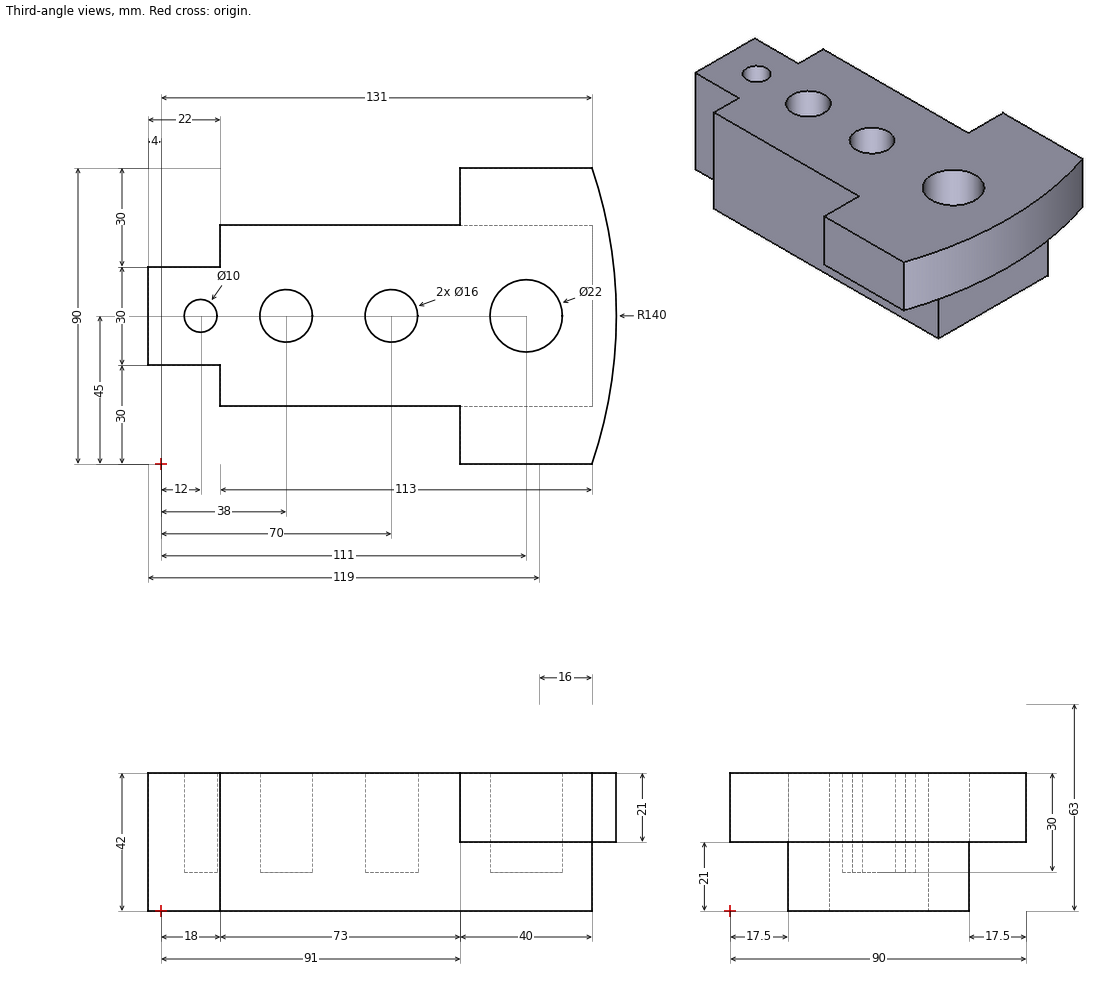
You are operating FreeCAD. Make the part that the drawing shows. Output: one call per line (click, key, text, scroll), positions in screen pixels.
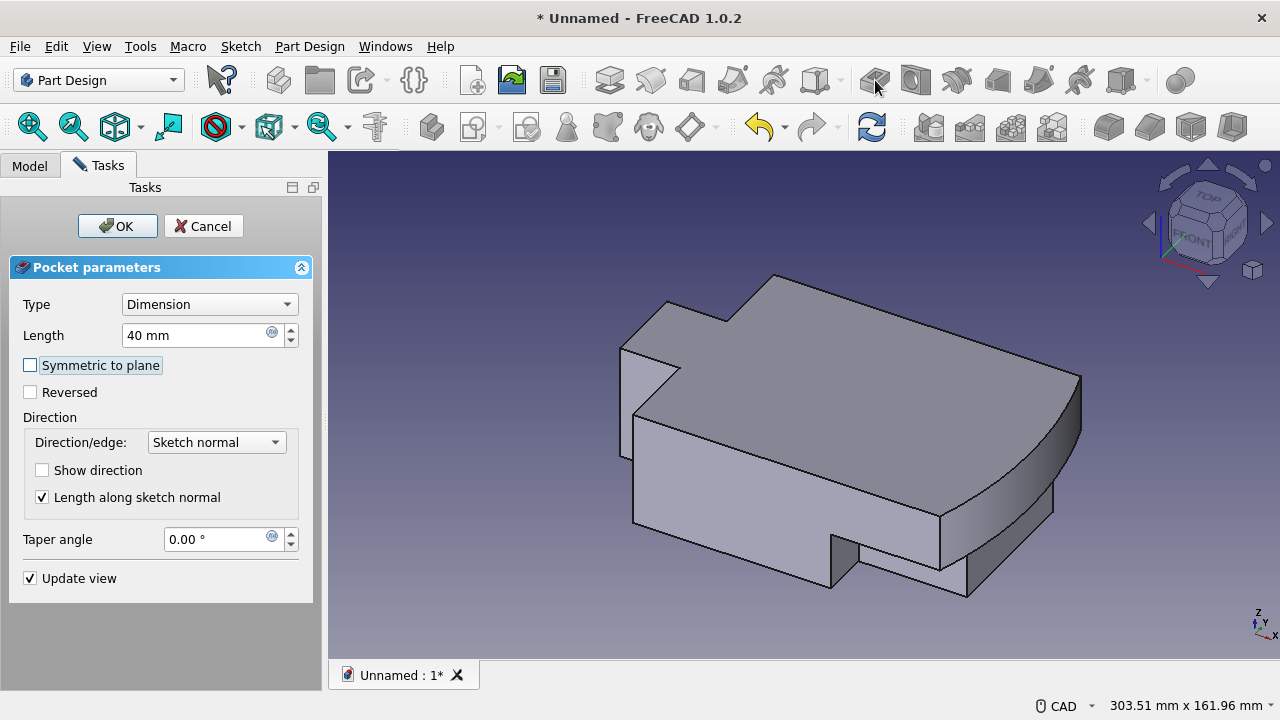
click(118, 226)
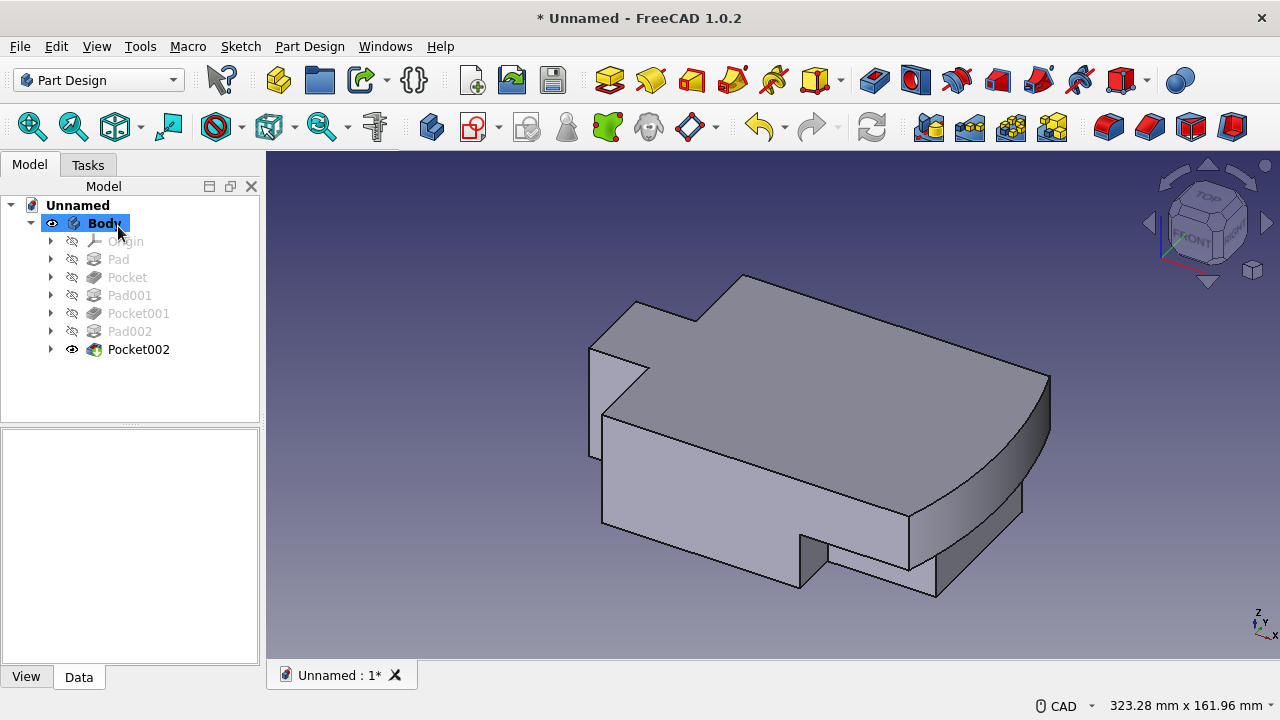
click(472, 128)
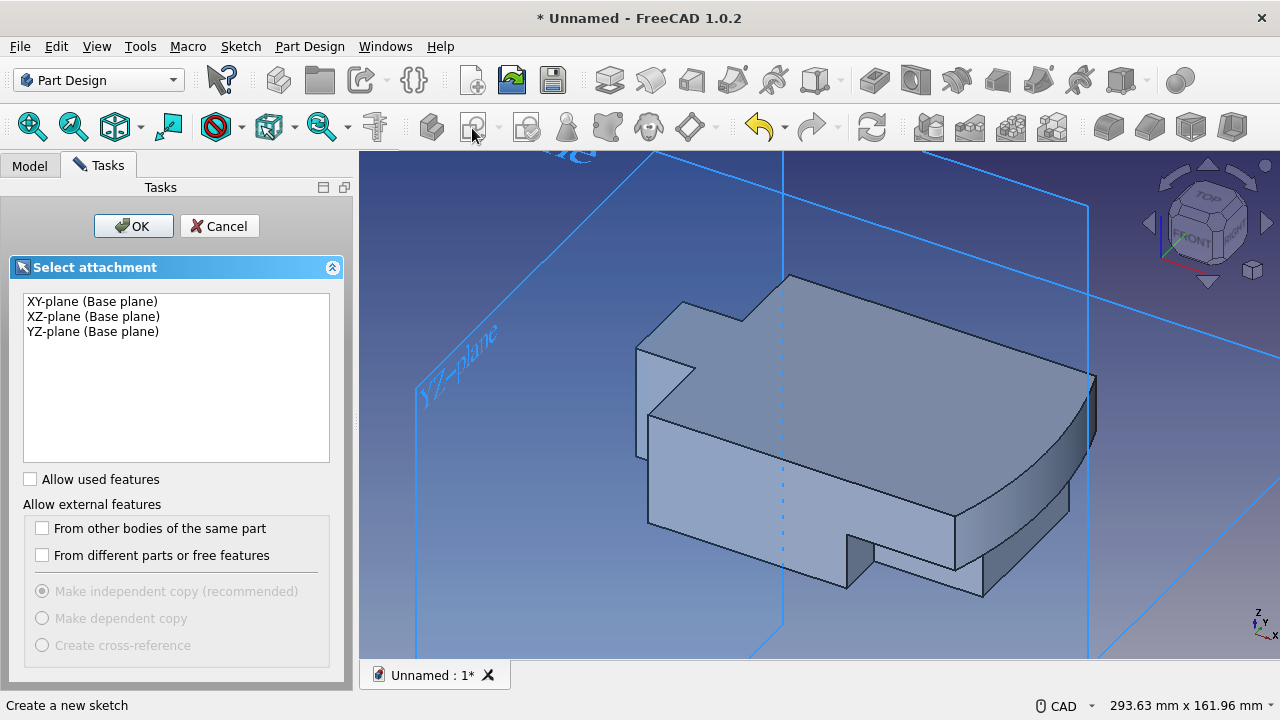
click(84, 316)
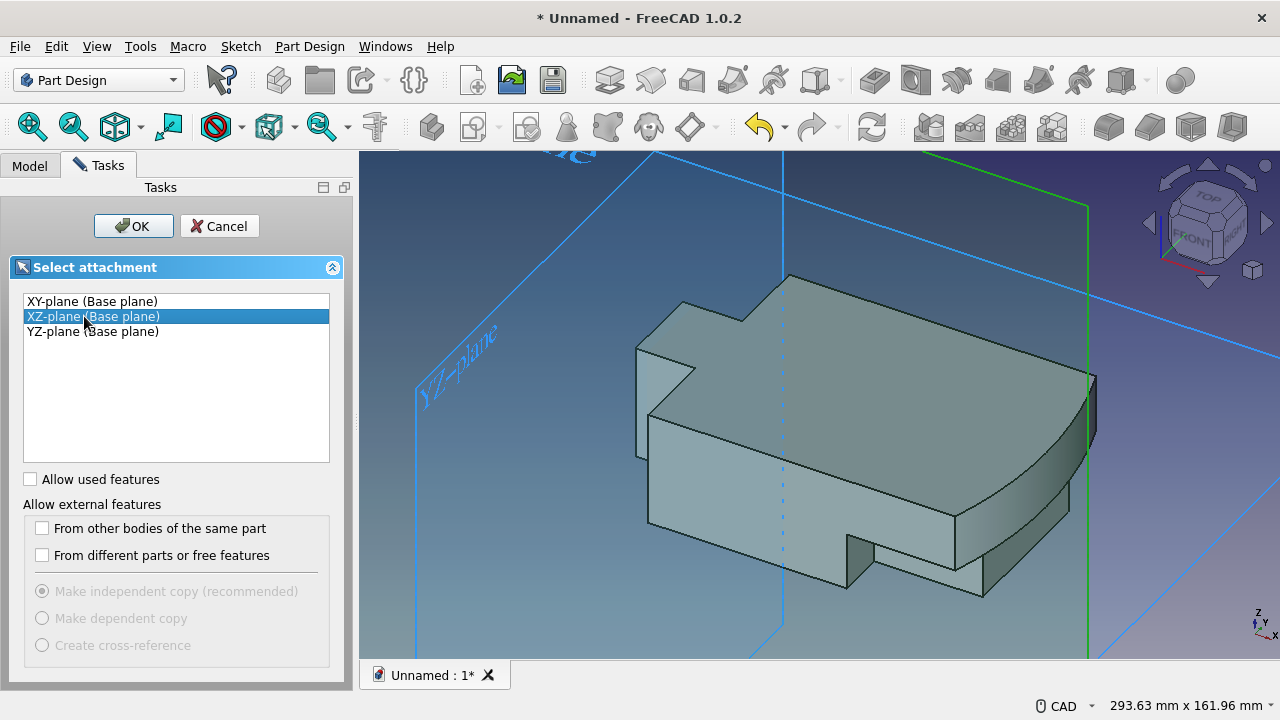
click(134, 226)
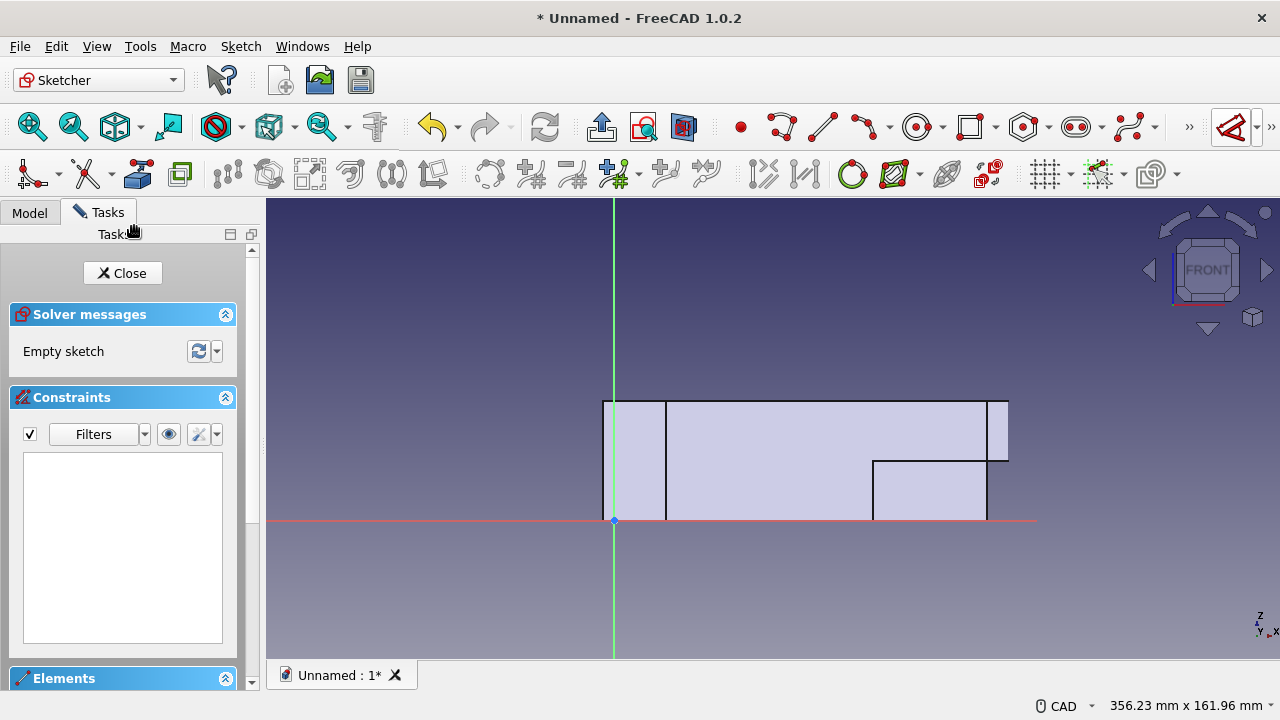
scroll(776, 488, up, 4)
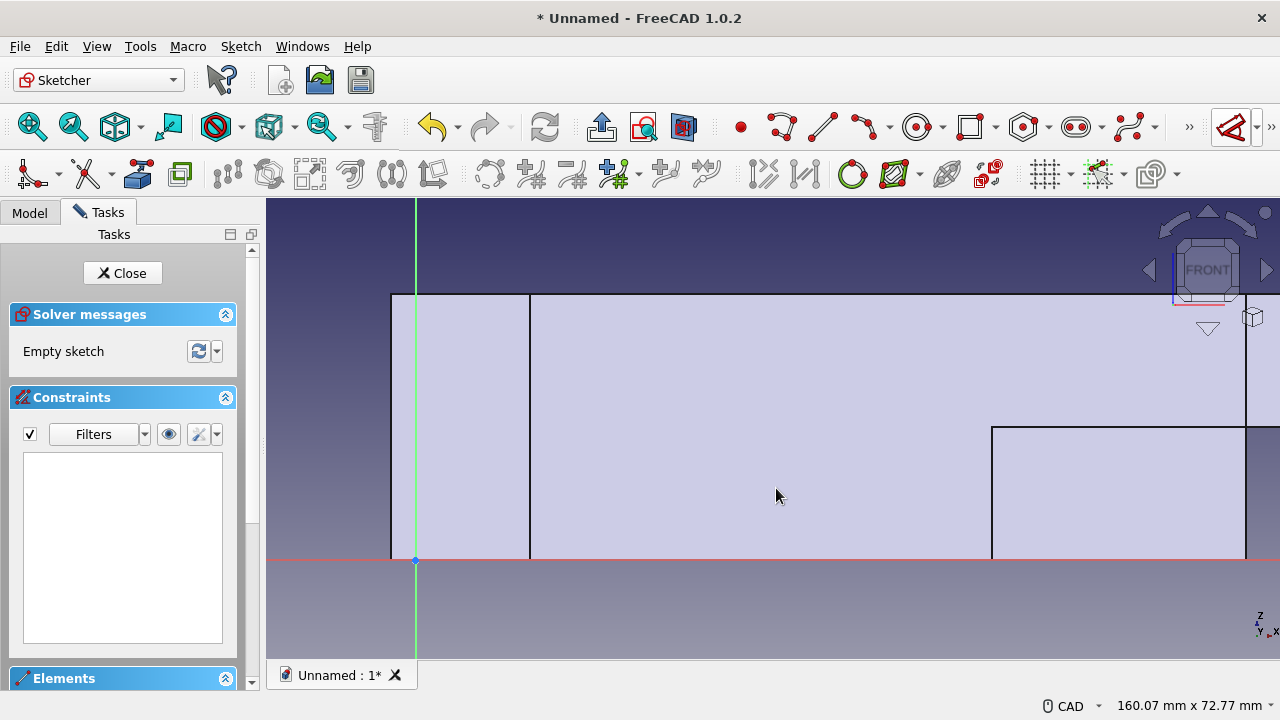
click(970, 128)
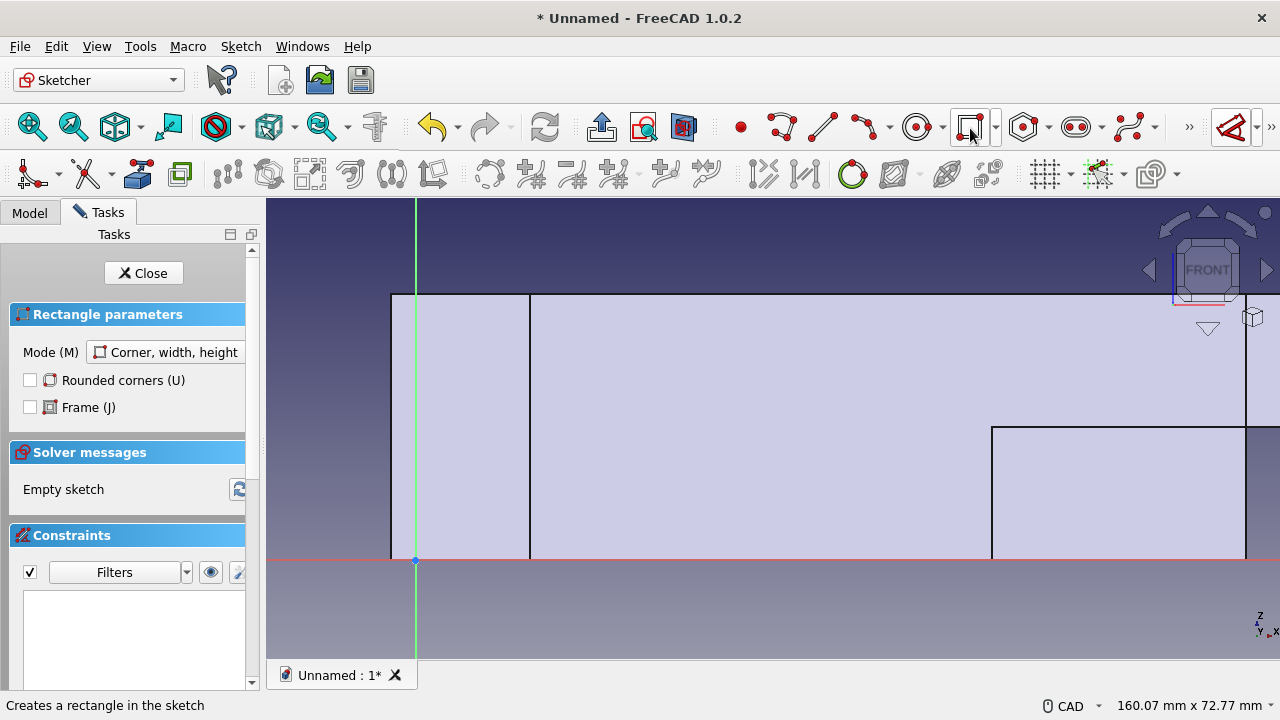
click(530, 294)
click(992, 560)
key(Escape)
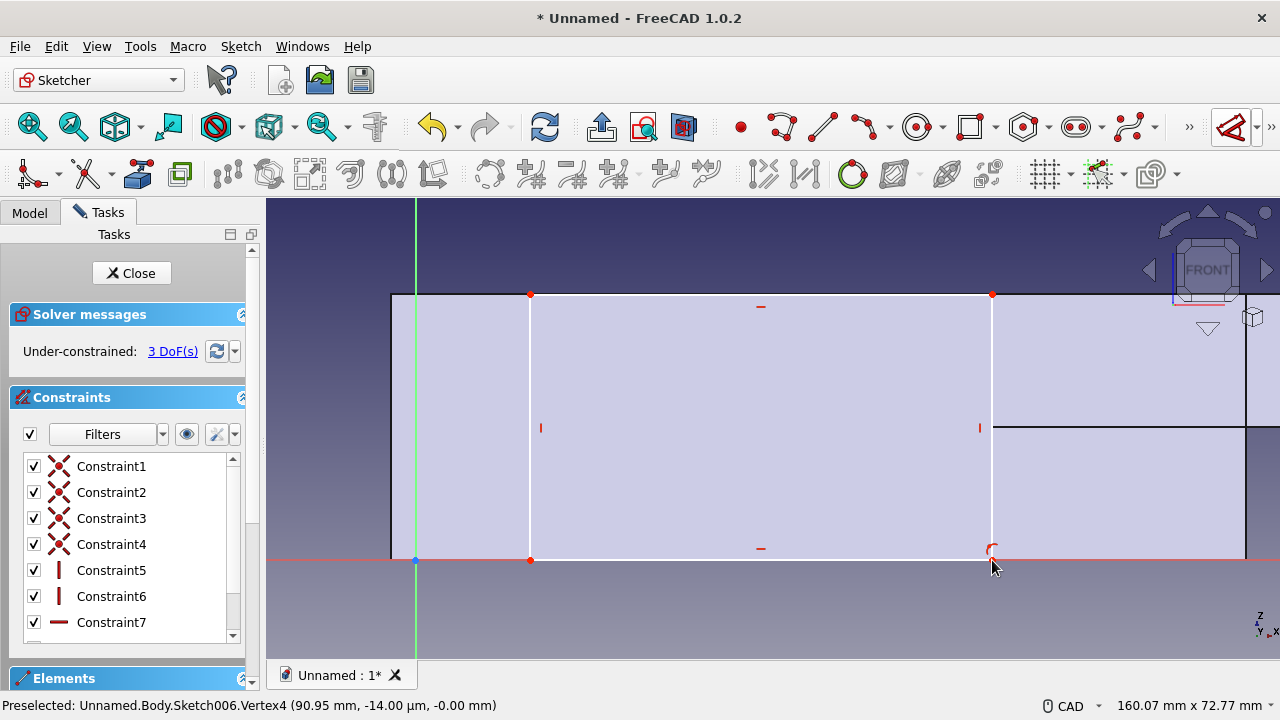
click(530, 375)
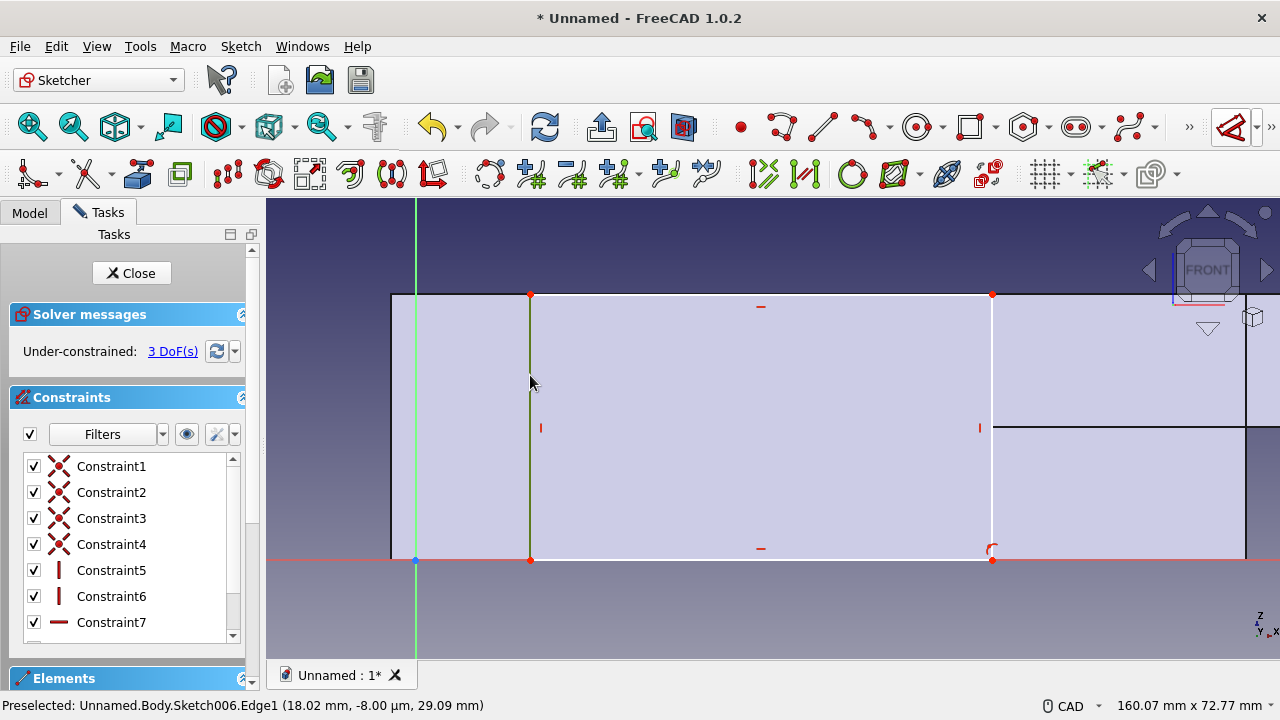
click(1256, 128)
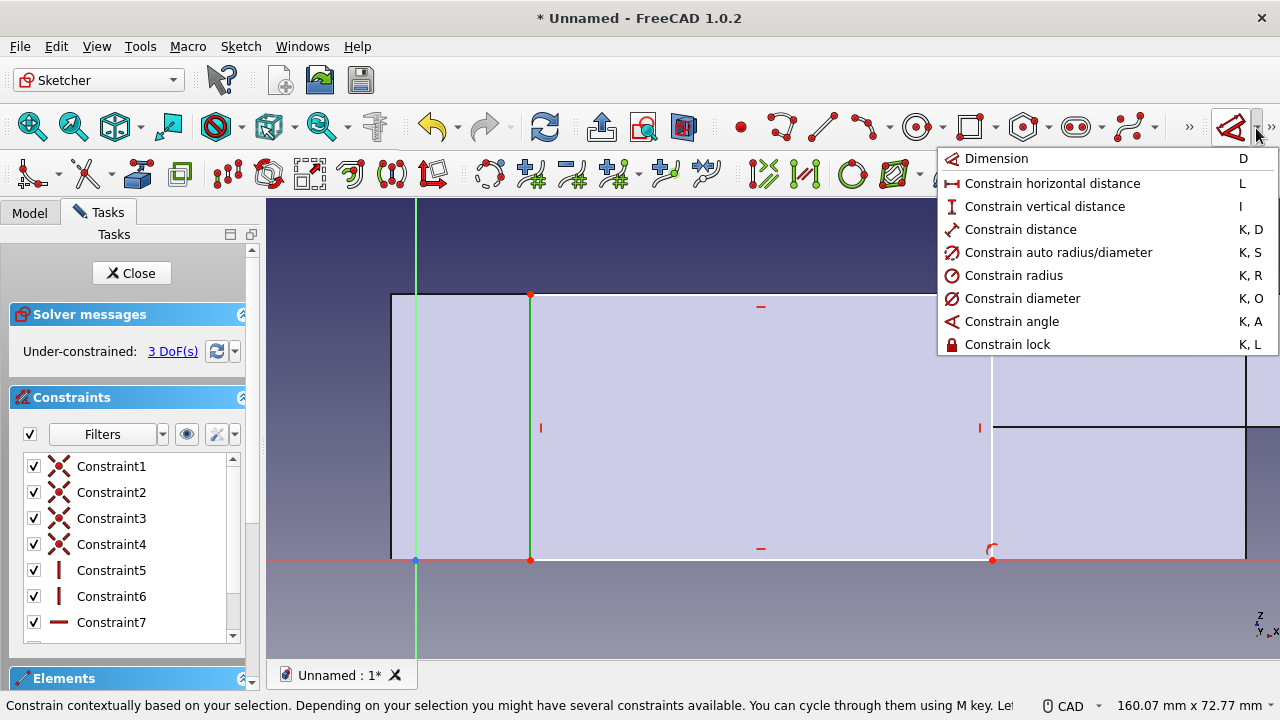
click(1108, 206)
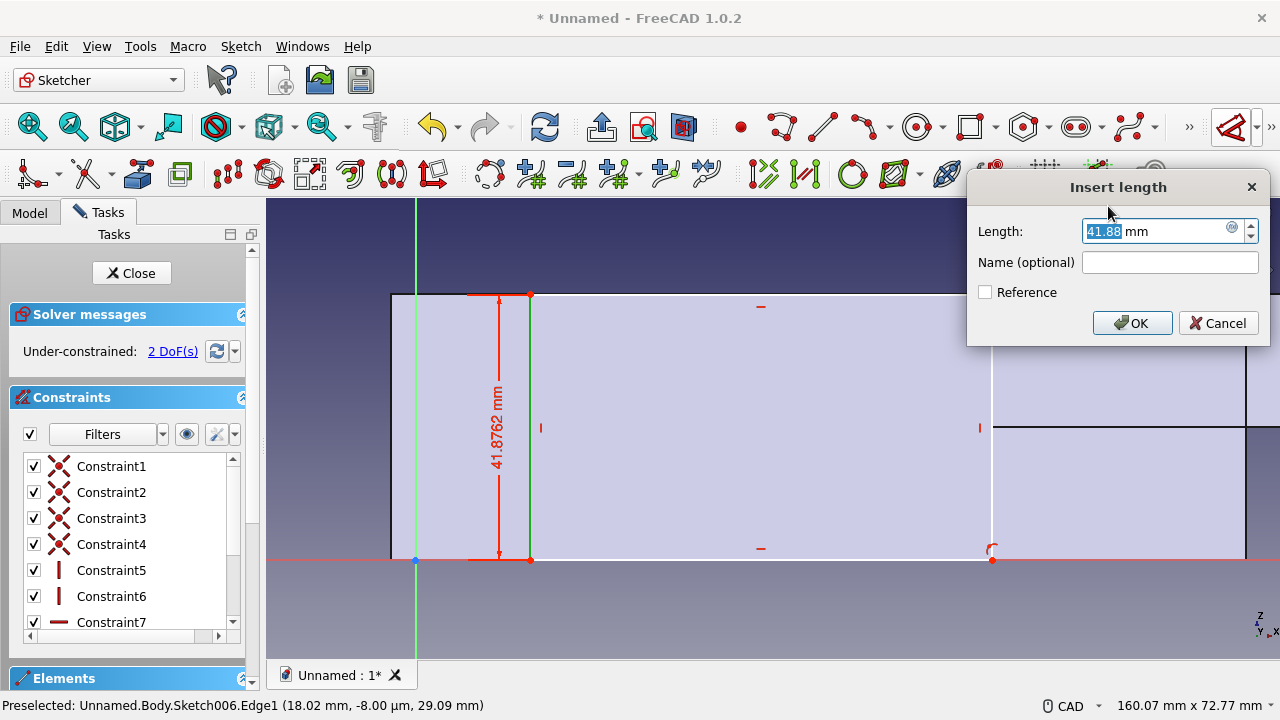
text(42)
key(Return)